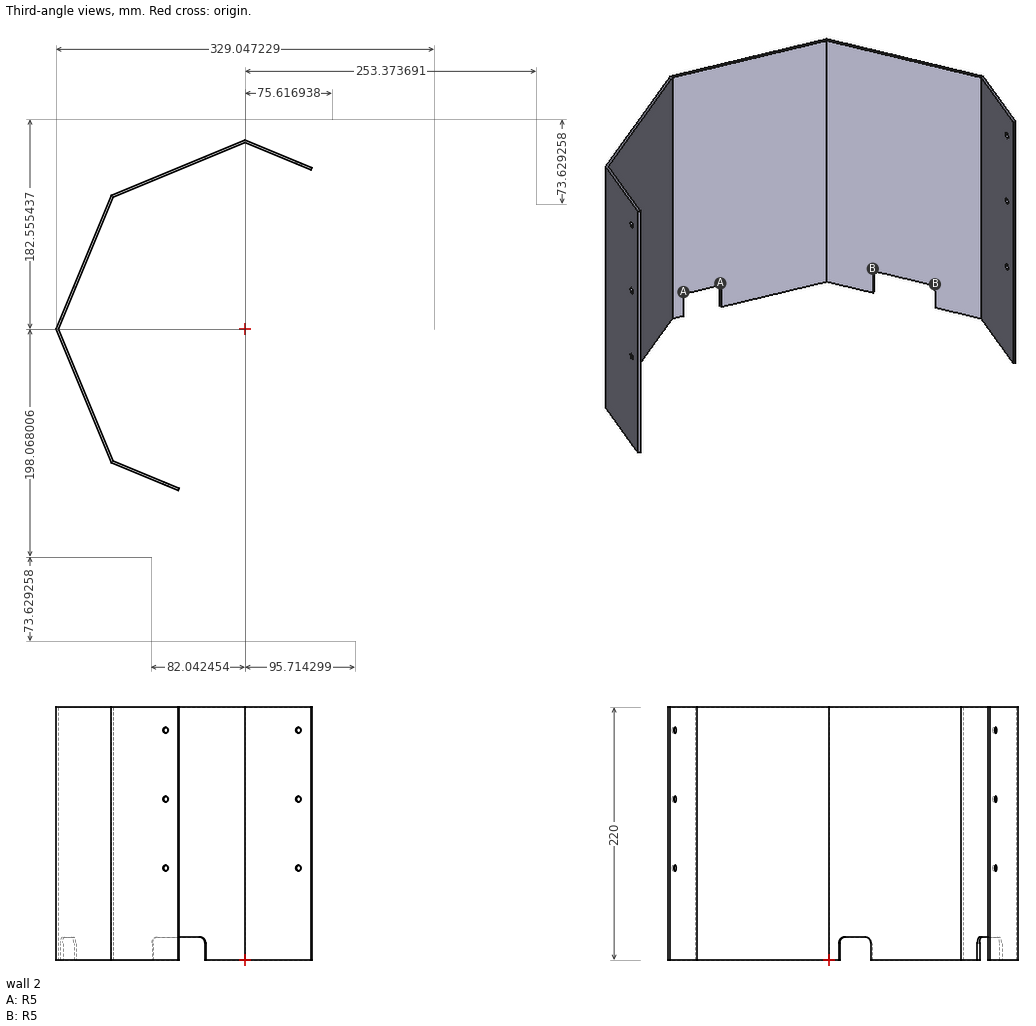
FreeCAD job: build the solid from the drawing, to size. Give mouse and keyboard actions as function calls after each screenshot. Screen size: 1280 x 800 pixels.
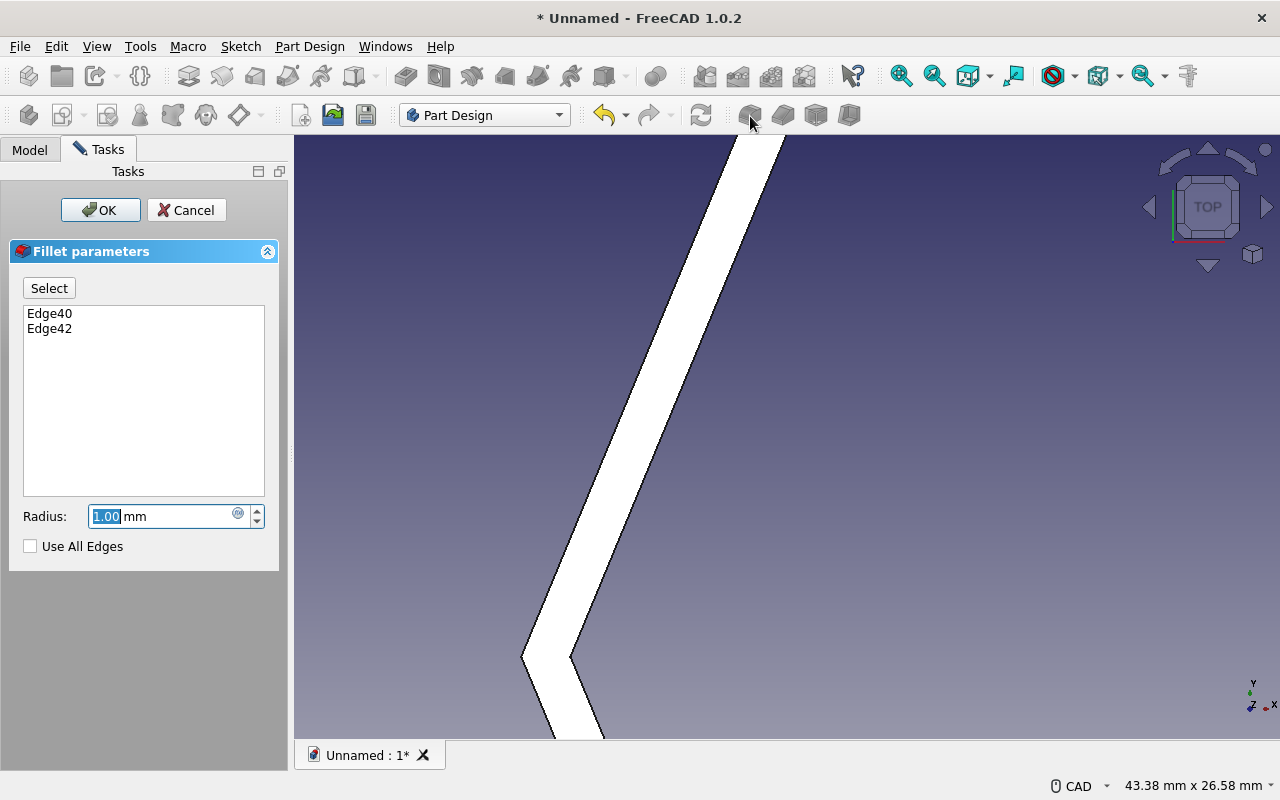
text(5)
key(Tab)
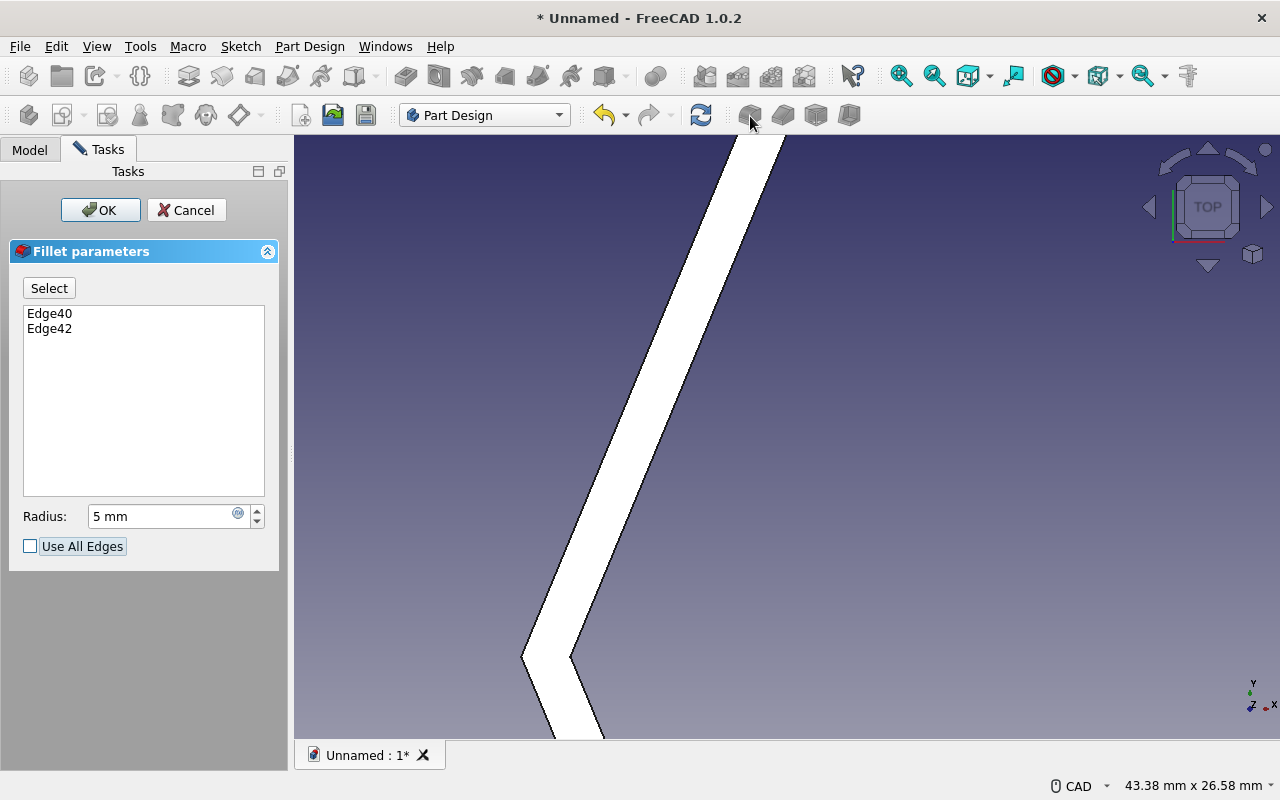
click(101, 210)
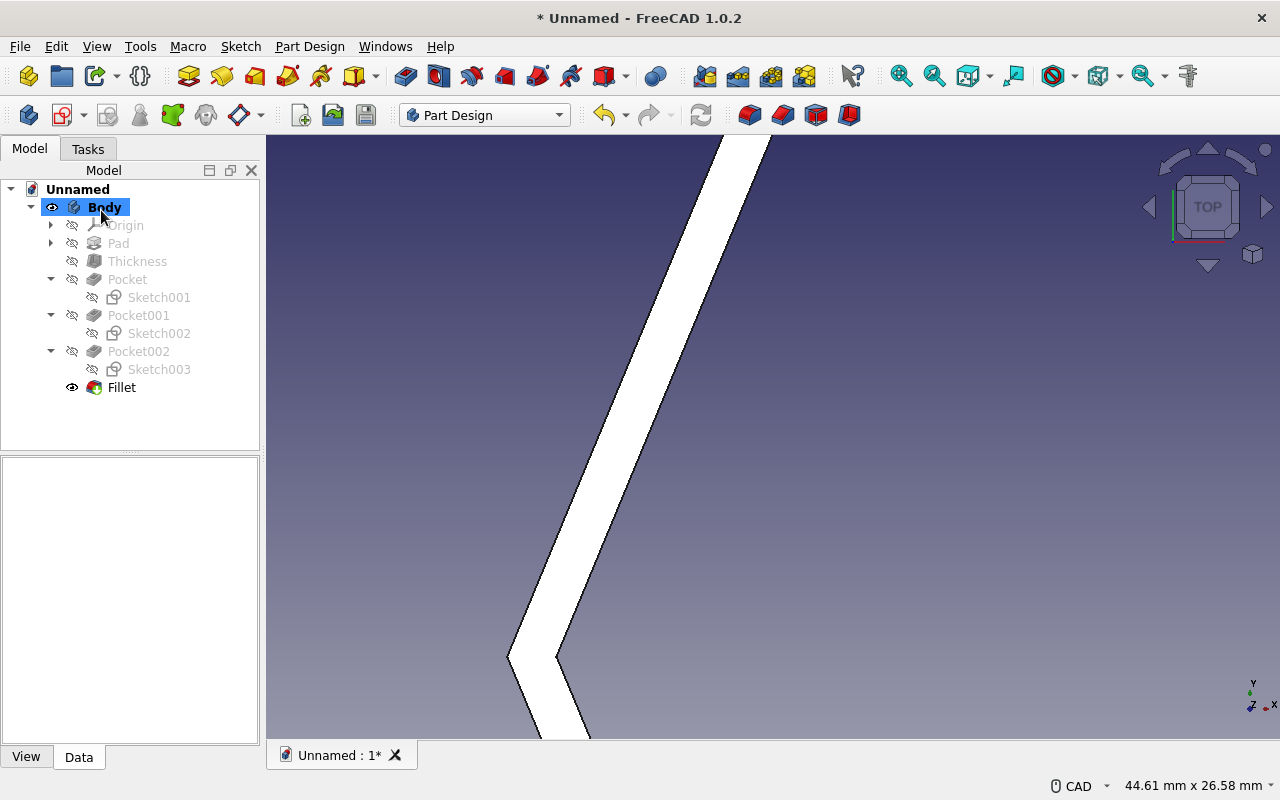
click(902, 76)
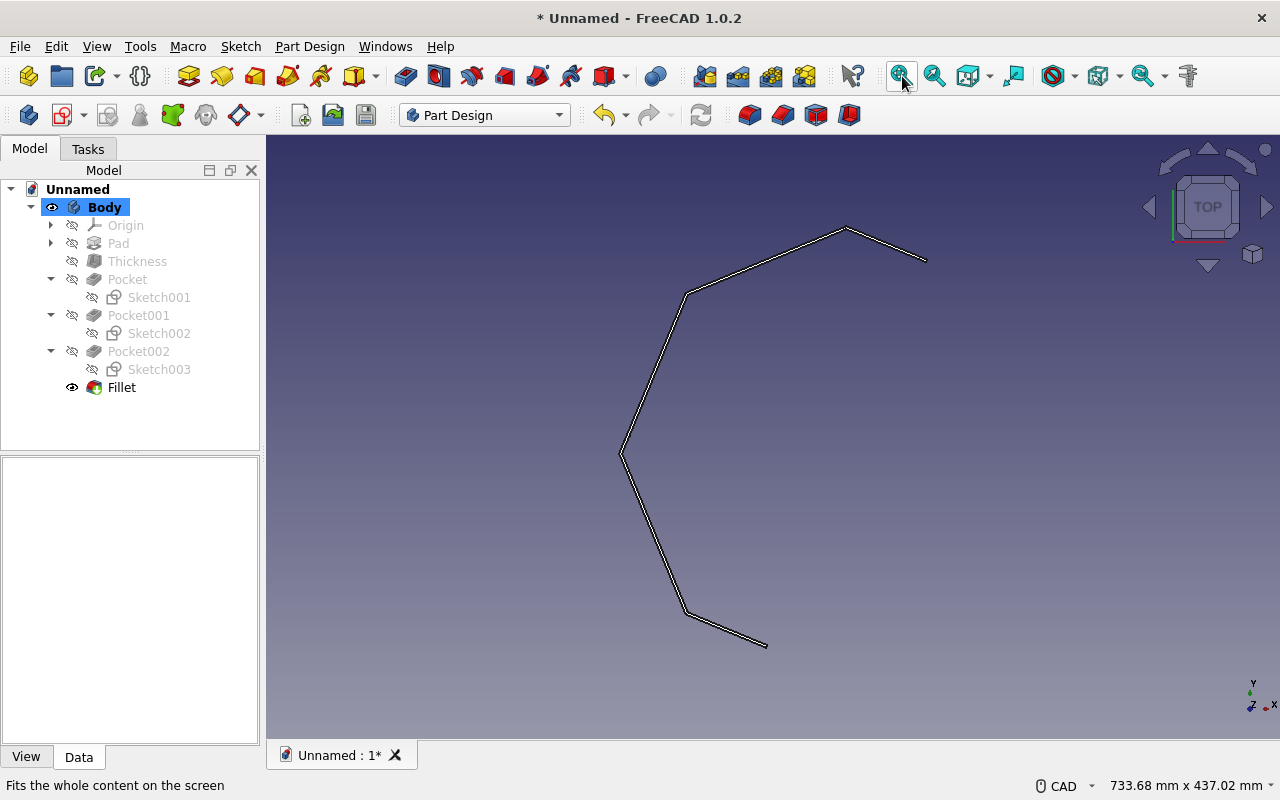
key(4)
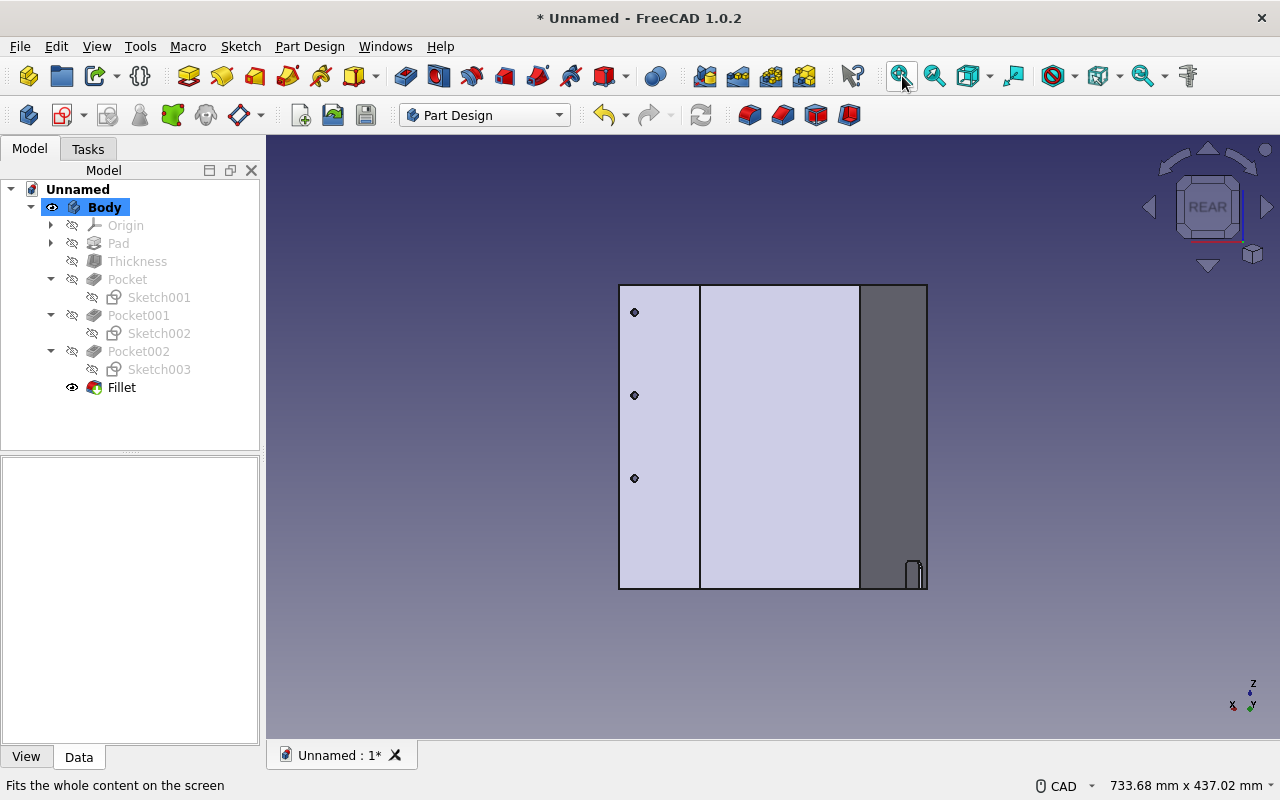
click(780, 393)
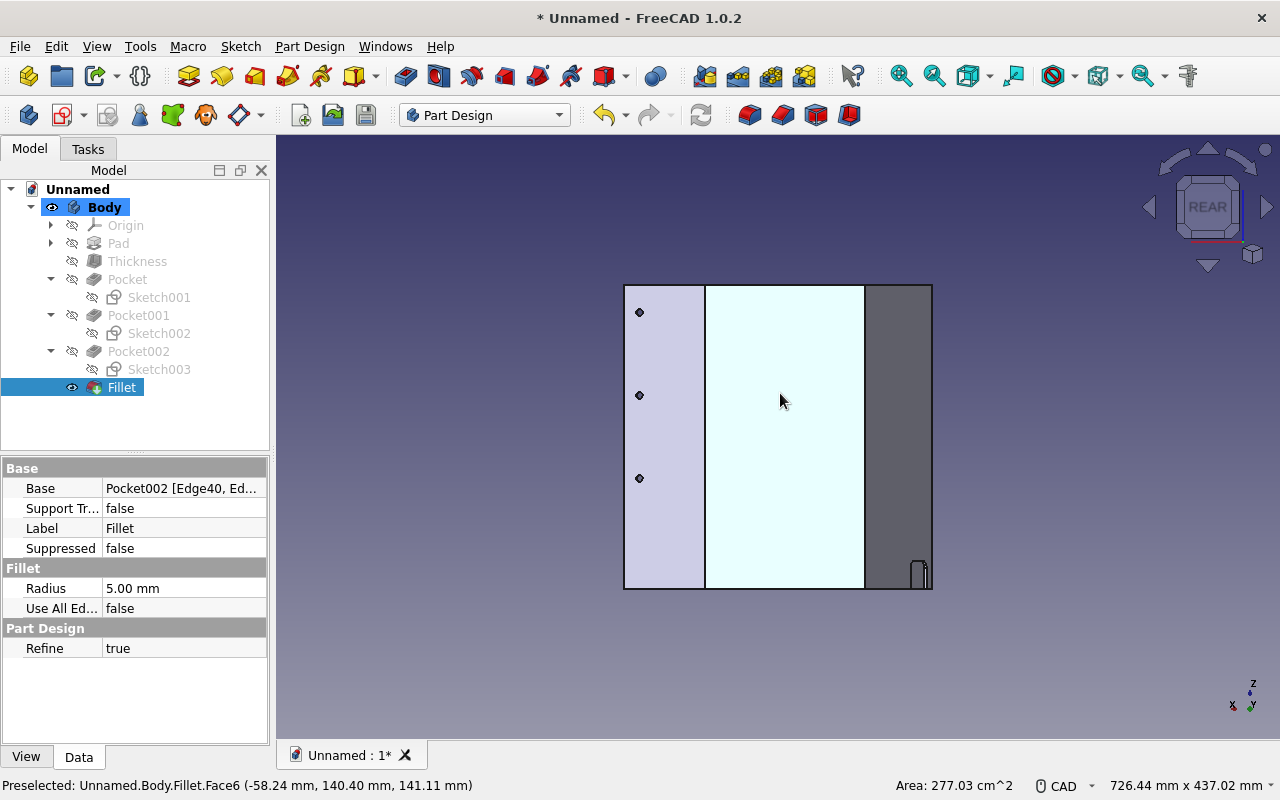
click(62, 116)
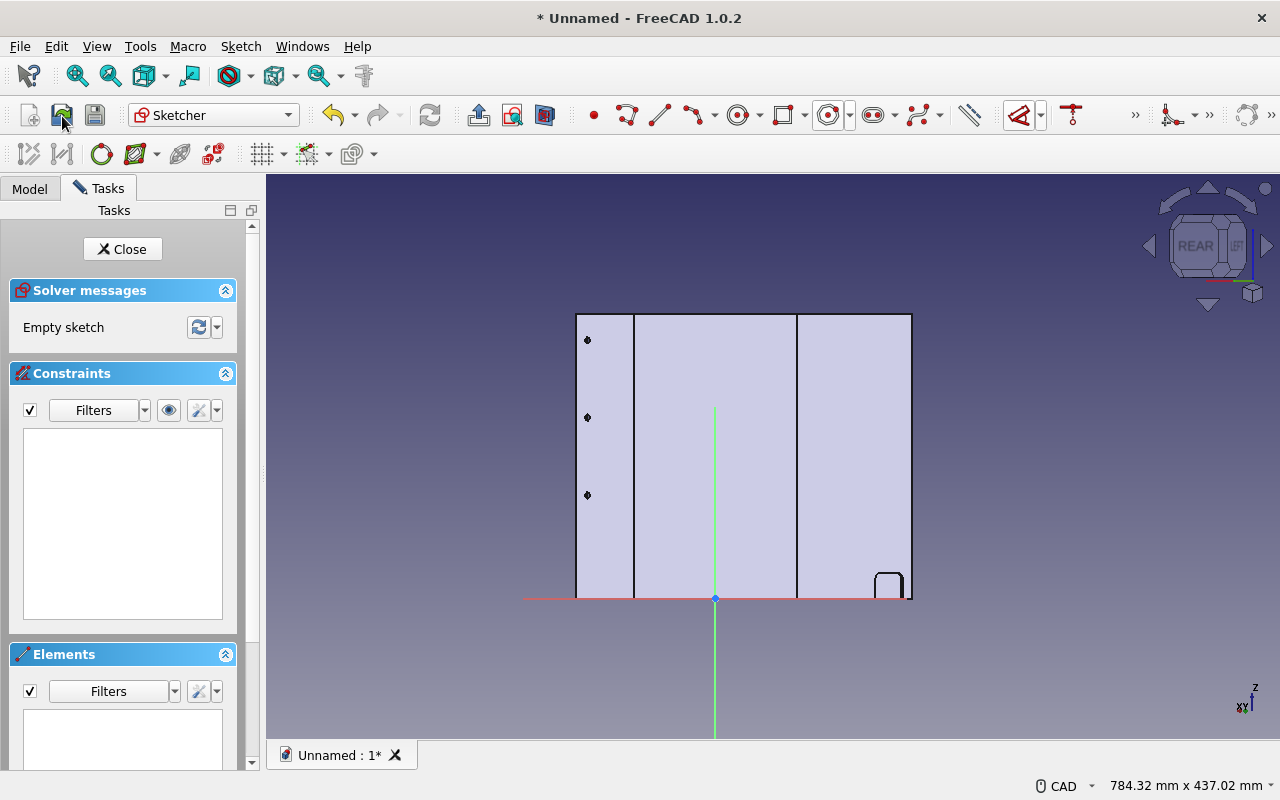
scroll(717, 602, up, 11)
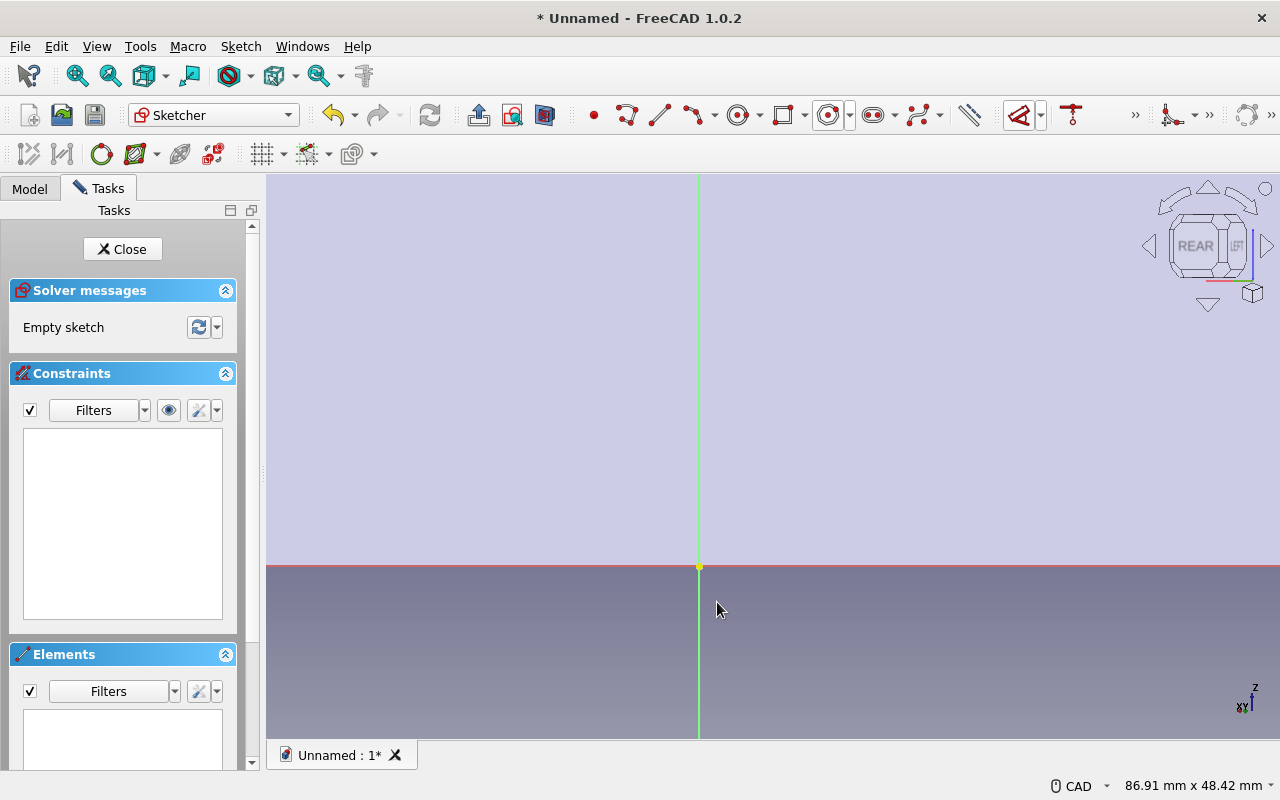
click(782, 116)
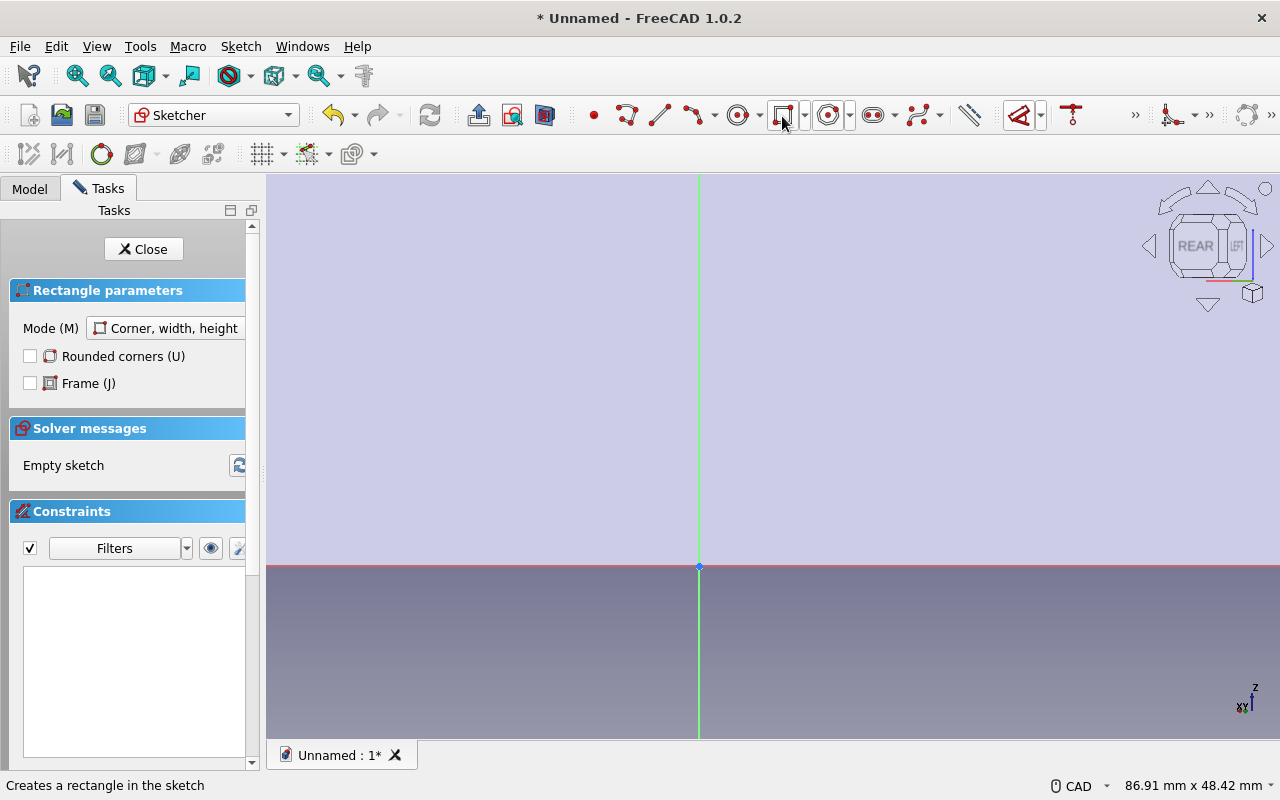
click(407, 333)
click(991, 566)
key(Escape)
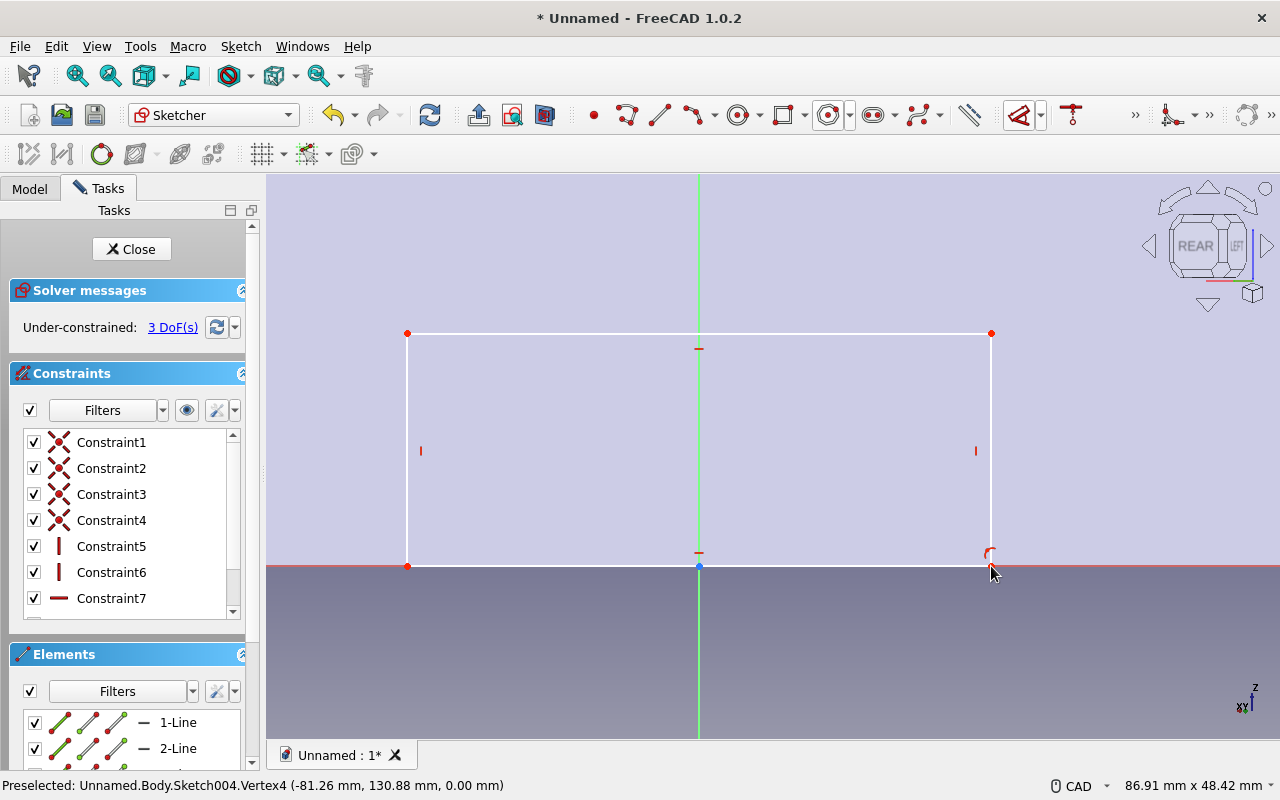
click(407, 404)